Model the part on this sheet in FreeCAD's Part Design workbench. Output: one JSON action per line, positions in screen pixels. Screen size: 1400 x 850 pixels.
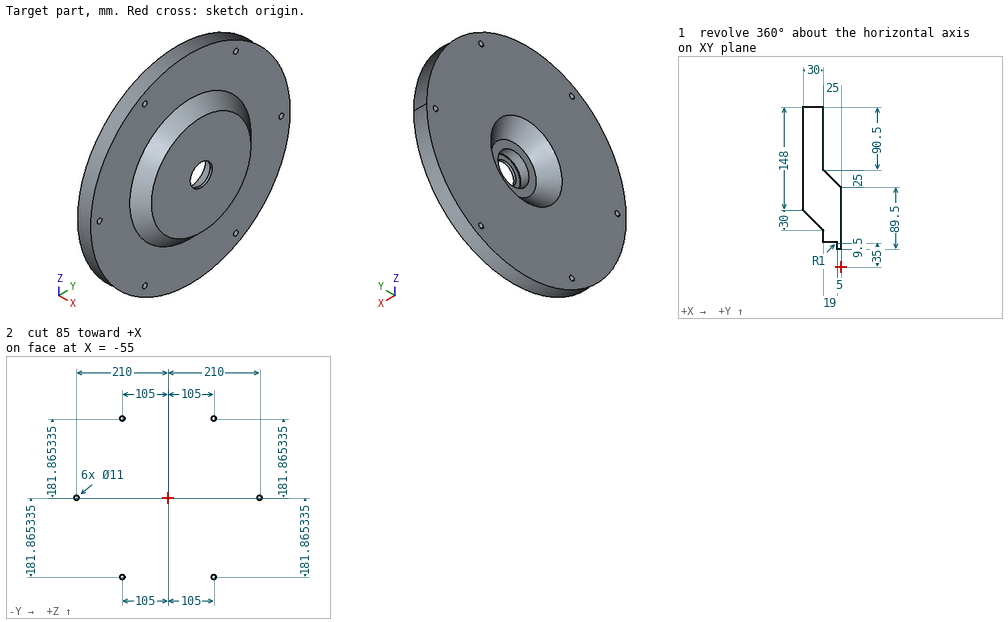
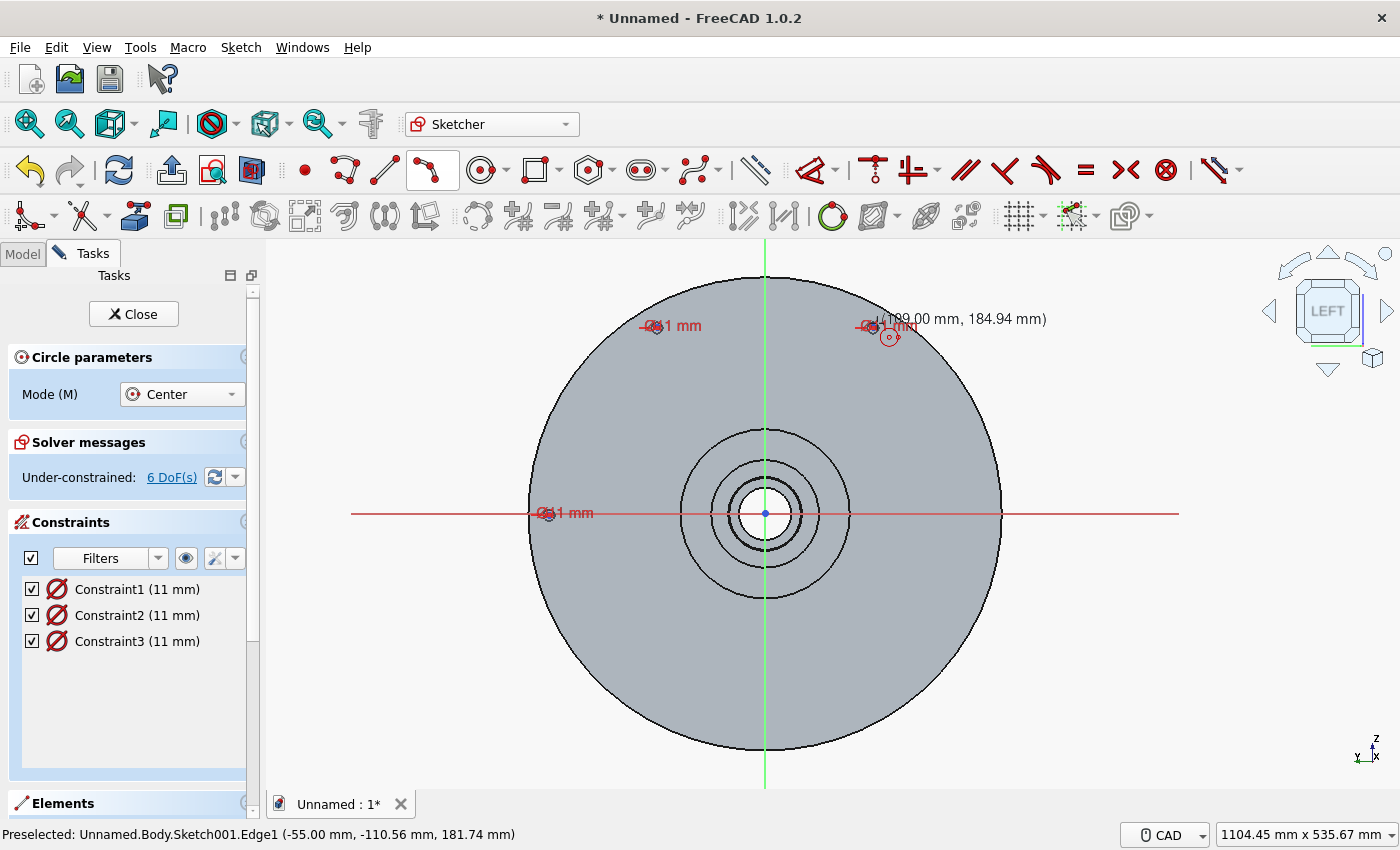
{"action": "scroll", "coordinate": [981, 514], "scroll_direction": "up", "scroll_amount": 7}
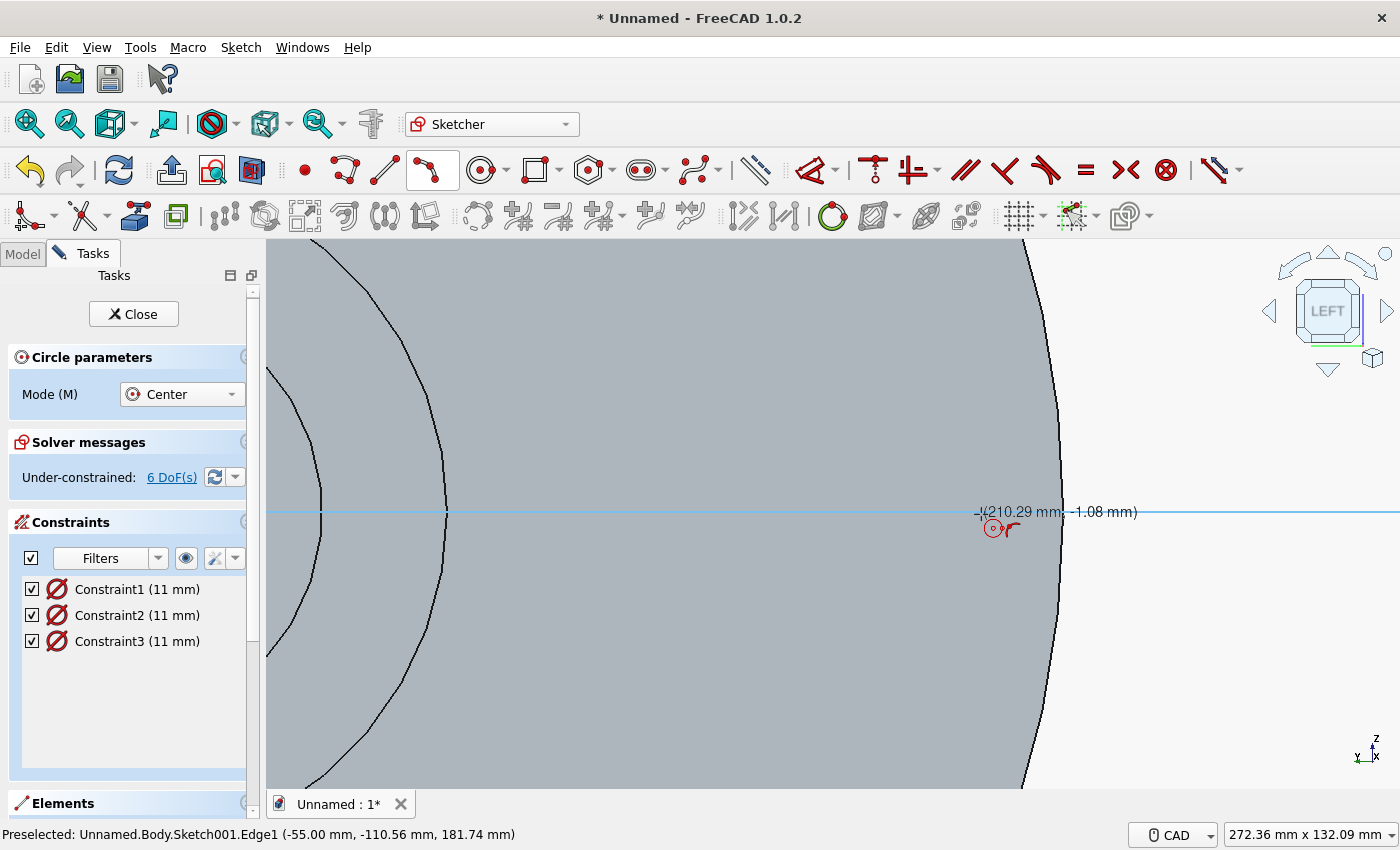
{"action": "scroll", "coordinate": [981, 515], "scroll_direction": "down", "scroll_amount": 7}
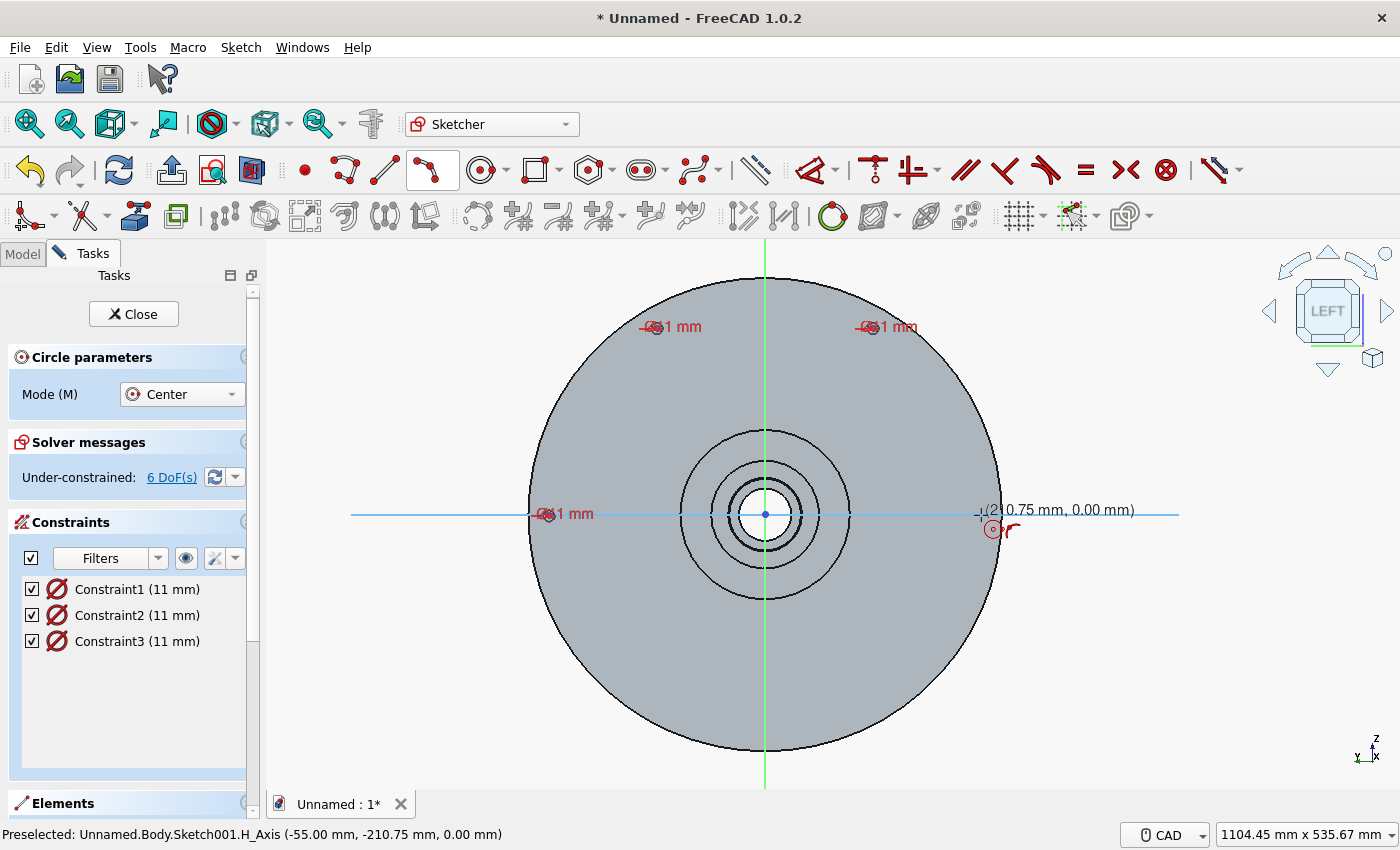
{"action": "left_click", "coordinate": [981, 515]}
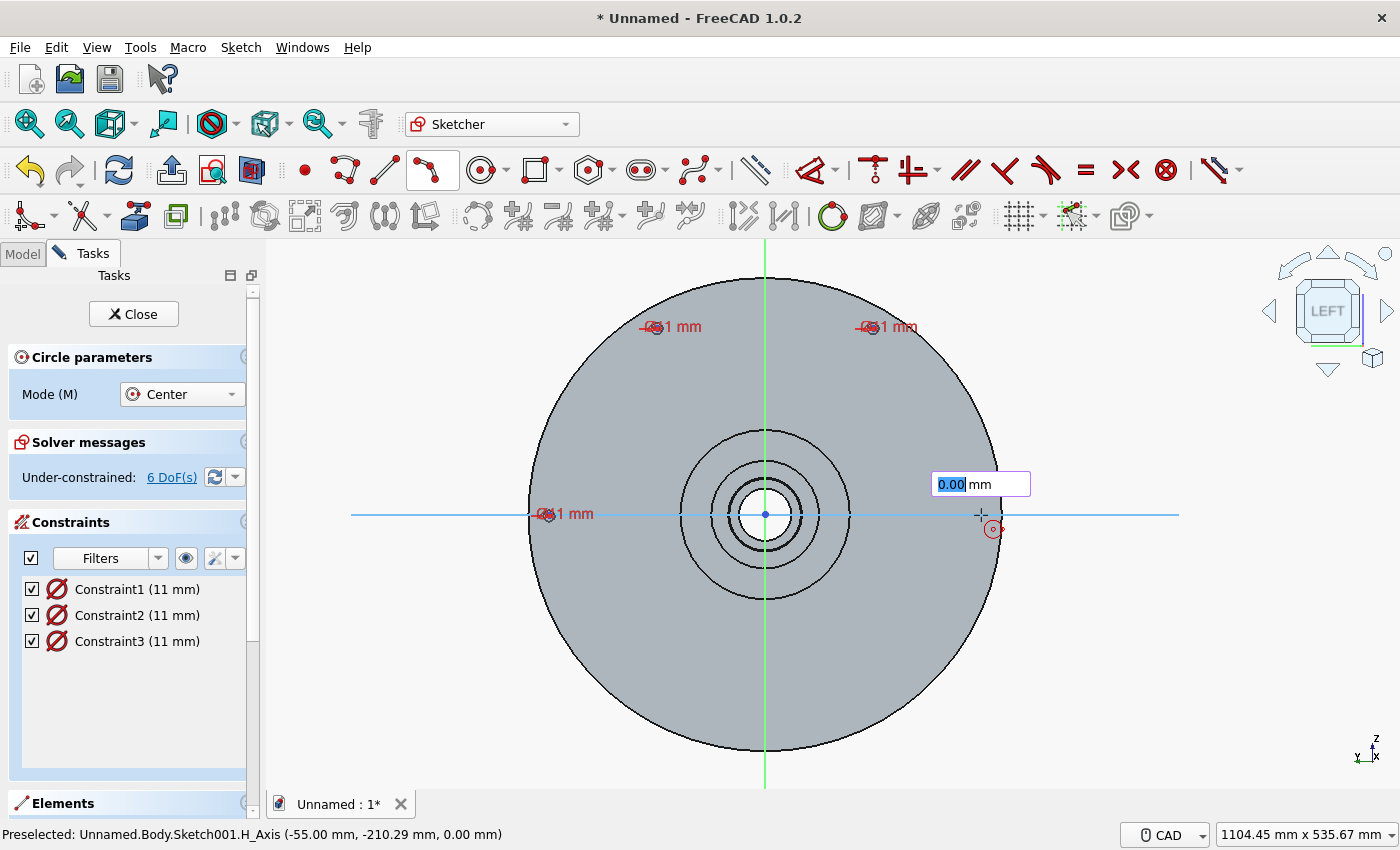
{"action": "scroll", "coordinate": [983, 509], "scroll_direction": "up", "scroll_amount": 6}
{"action": "mouse_move", "coordinate": [980, 509]}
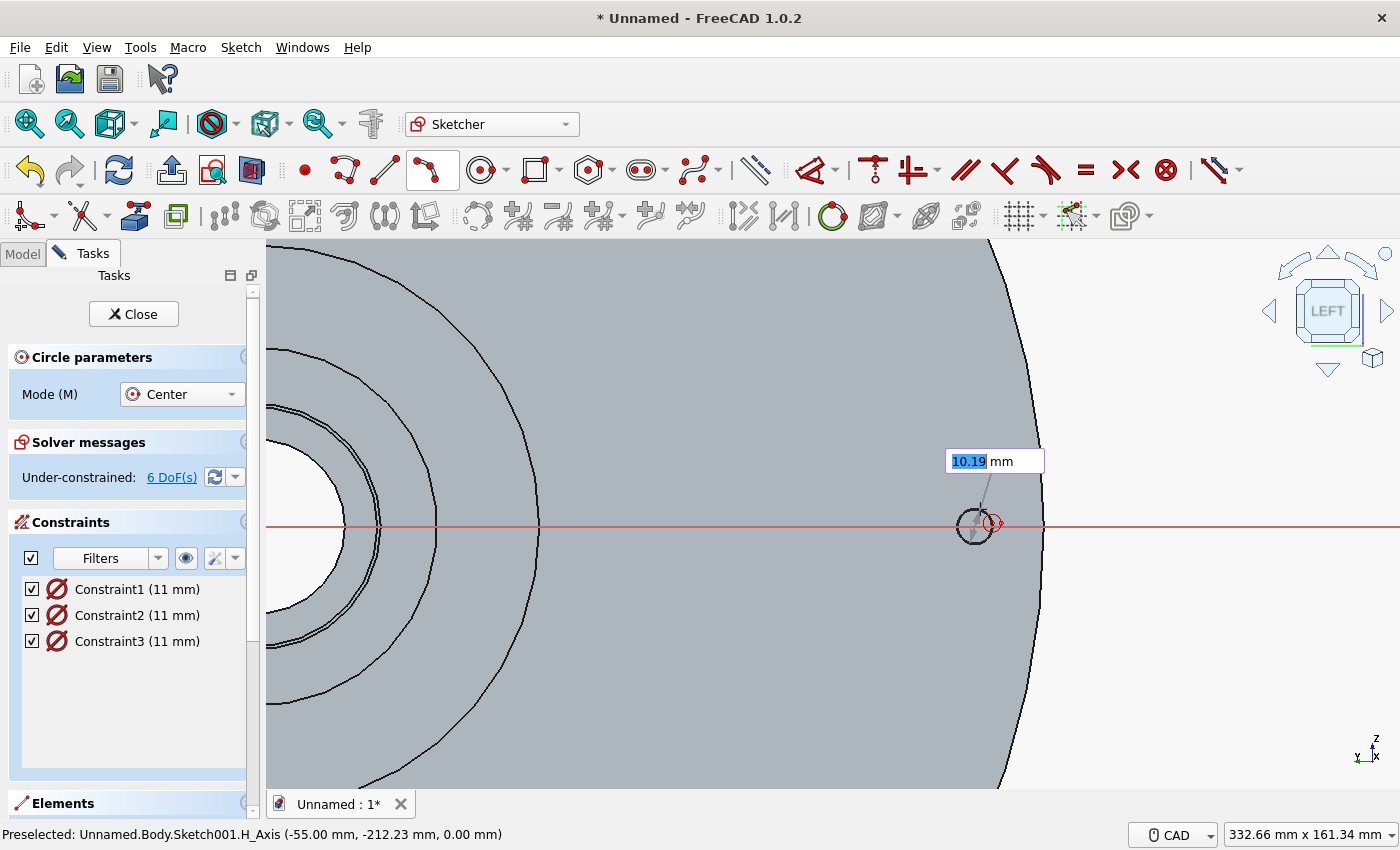
{"action": "type", "text": "11"}
{"action": "key", "text": "Return"}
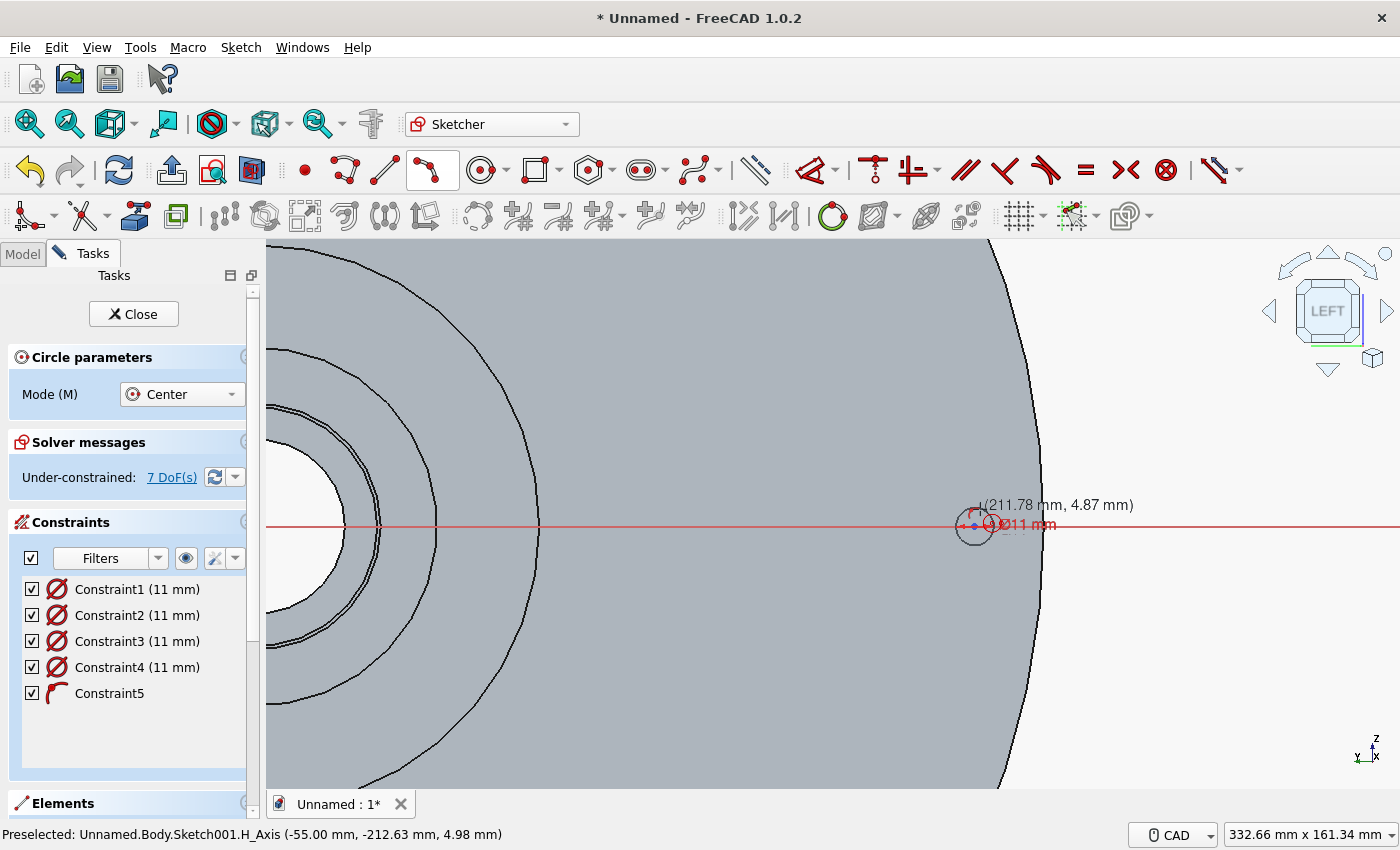
{"action": "scroll", "coordinate": [983, 509], "scroll_direction": "down", "scroll_amount": 6}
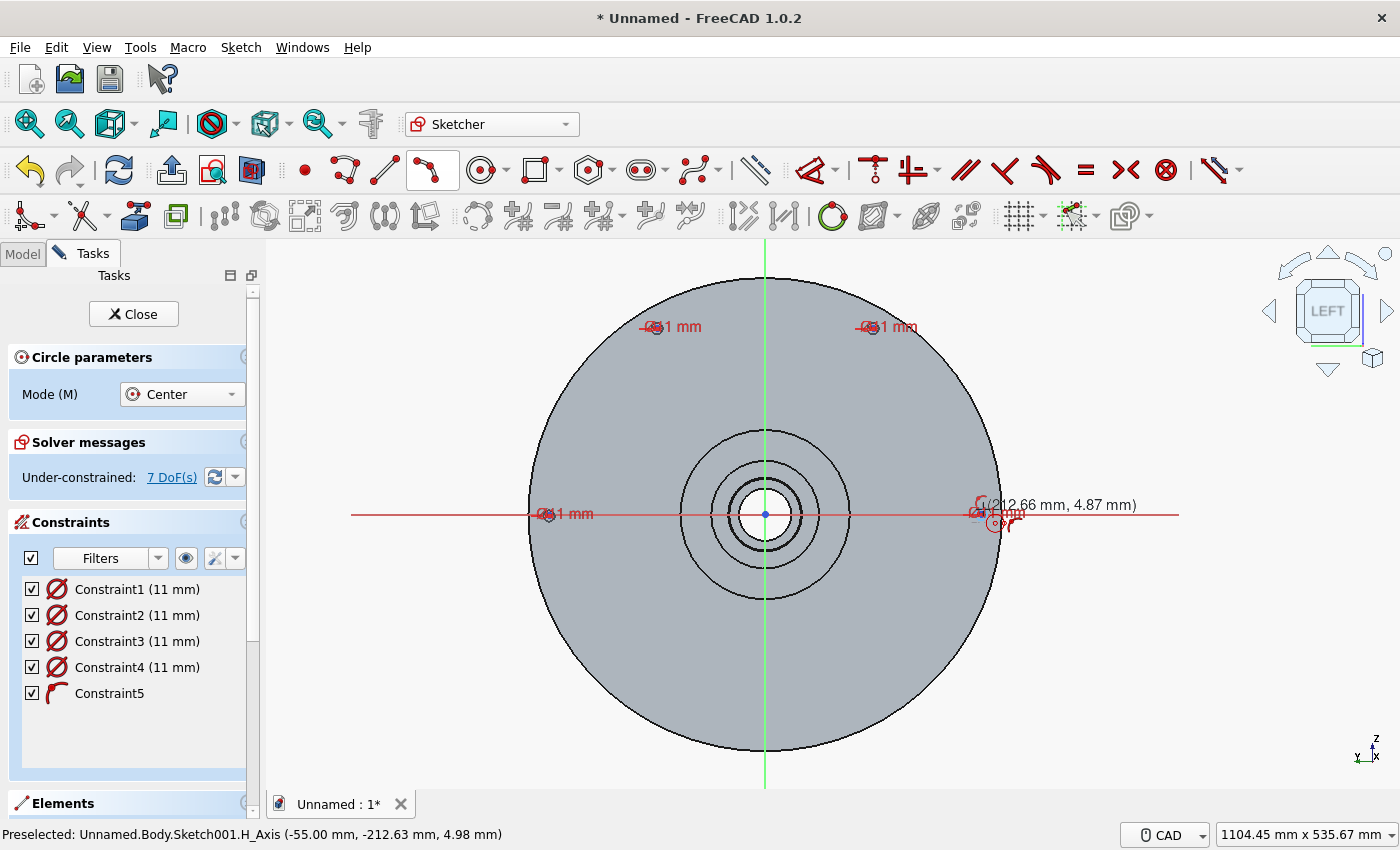
{"action": "scroll", "coordinate": [873, 701], "scroll_direction": "up", "scroll_amount": 7}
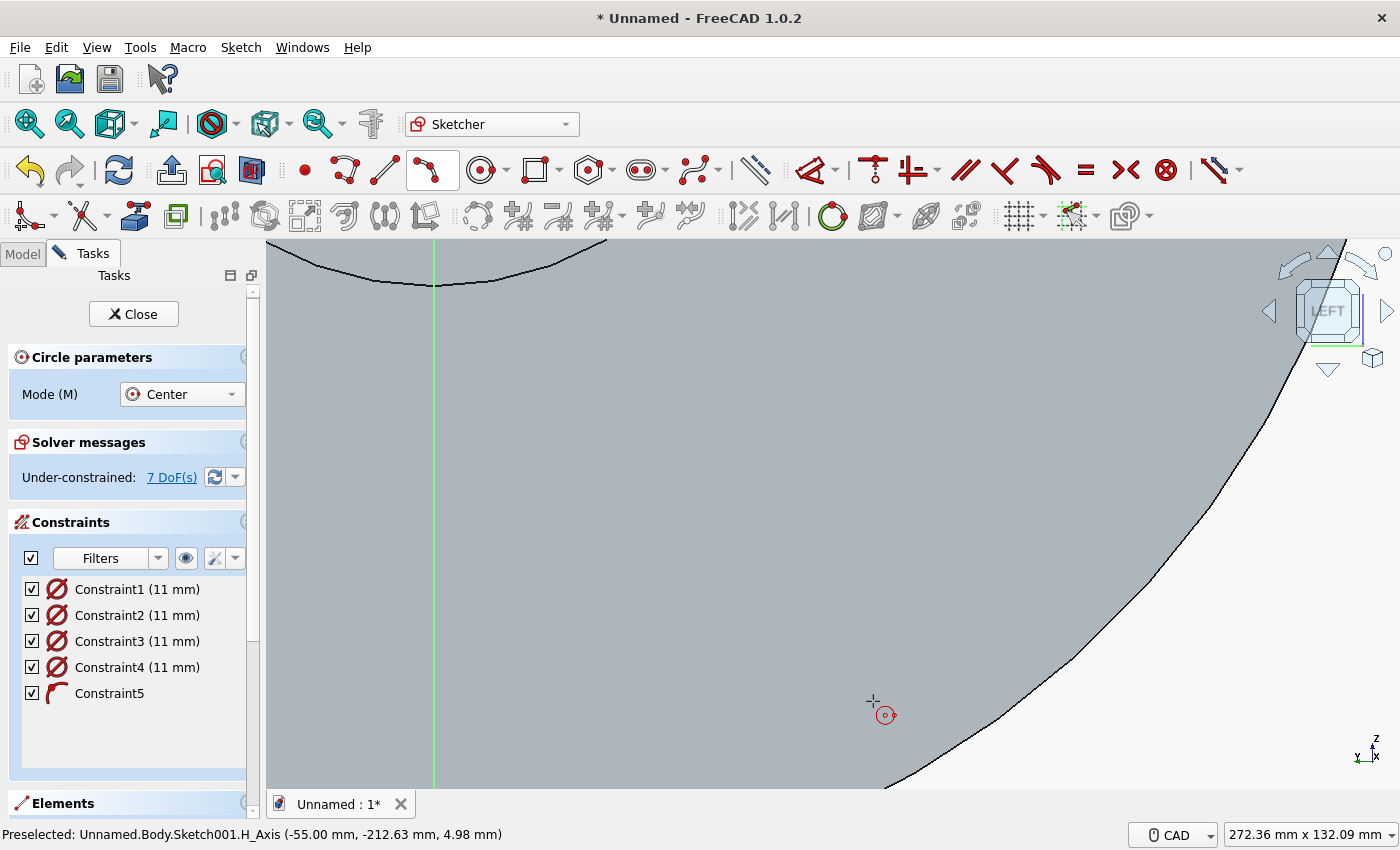
{"action": "scroll", "coordinate": [873, 701], "scroll_direction": "down", "scroll_amount": 7}